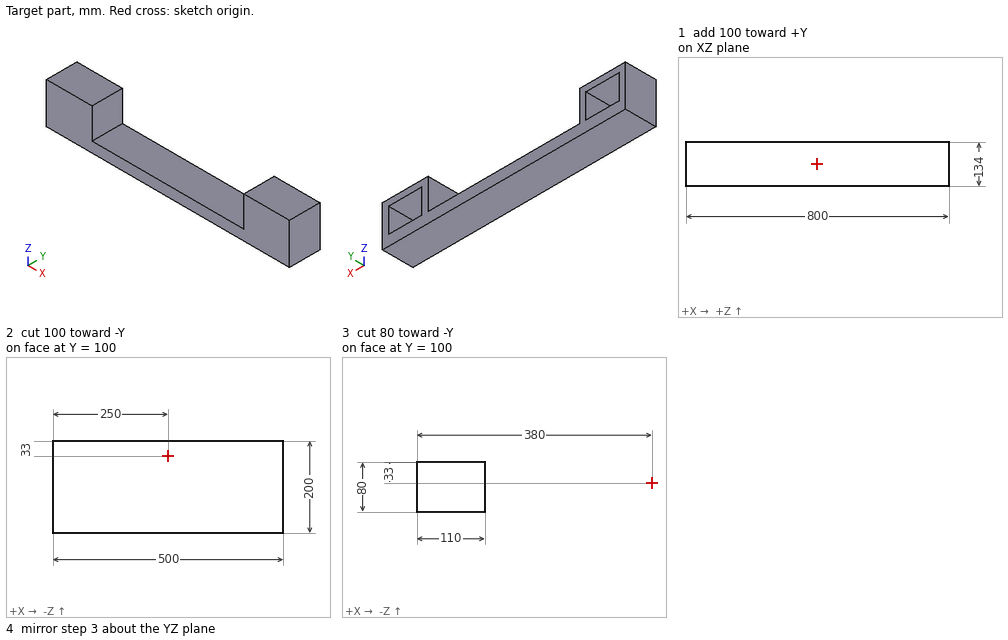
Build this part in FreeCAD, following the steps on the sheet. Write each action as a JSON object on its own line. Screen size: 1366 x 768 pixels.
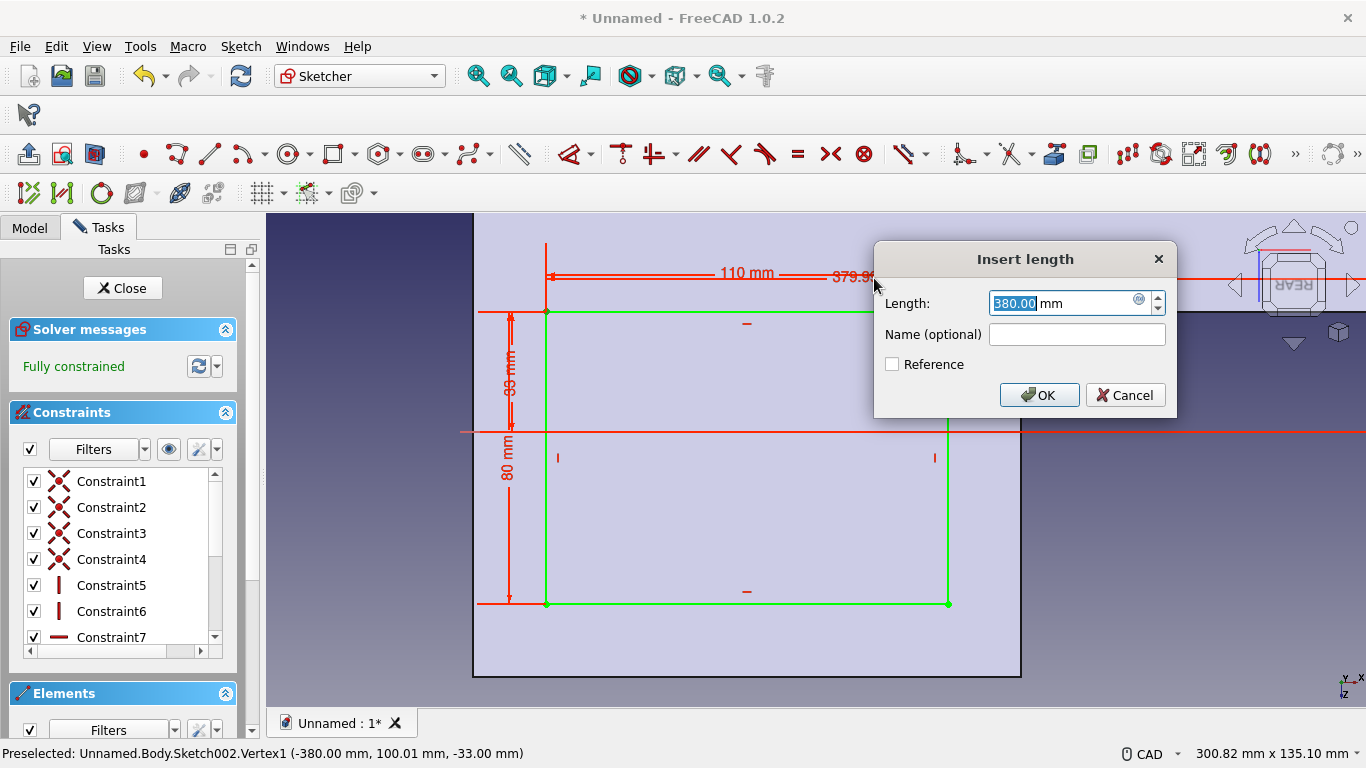
{"action": "type", "text": "380"}
{"action": "key", "text": "Return"}
{"action": "key", "text": "Escape"}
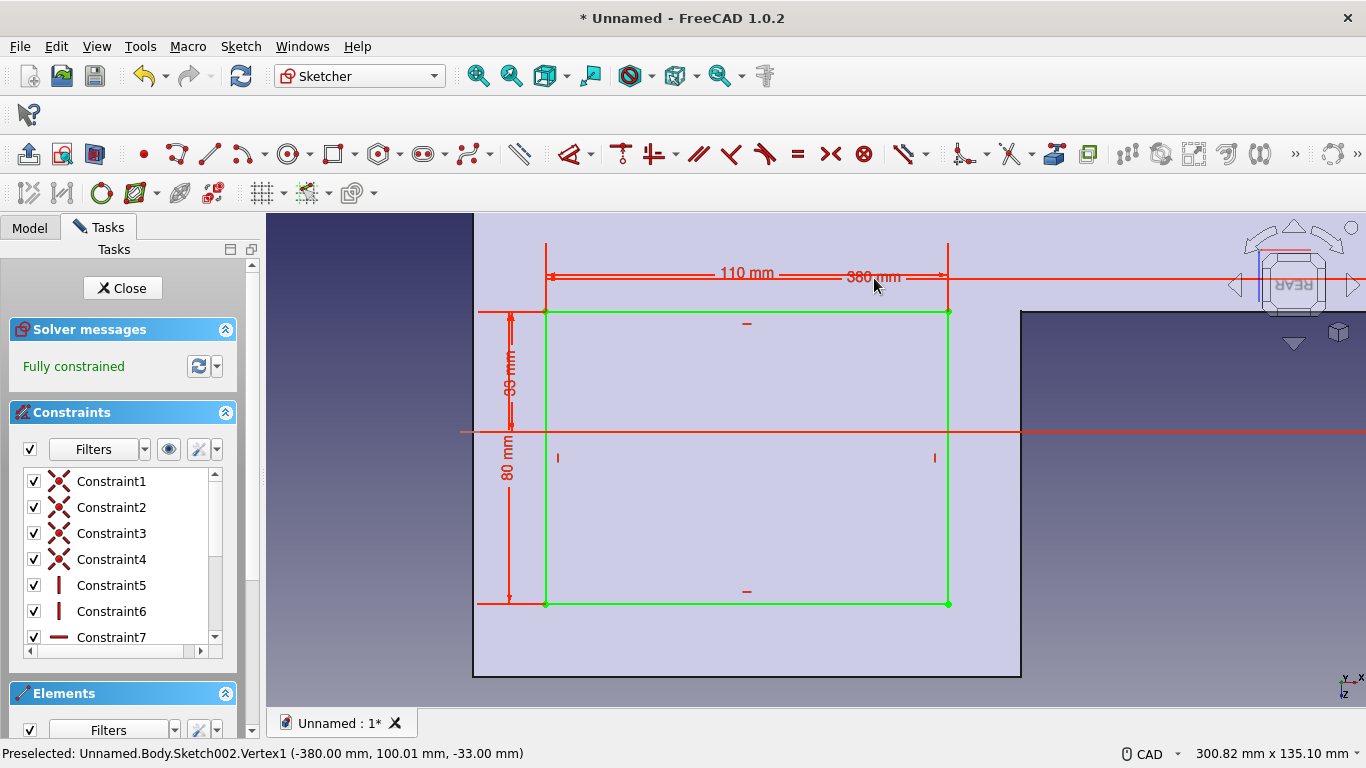
{"action": "left_click", "coordinate": [123, 288]}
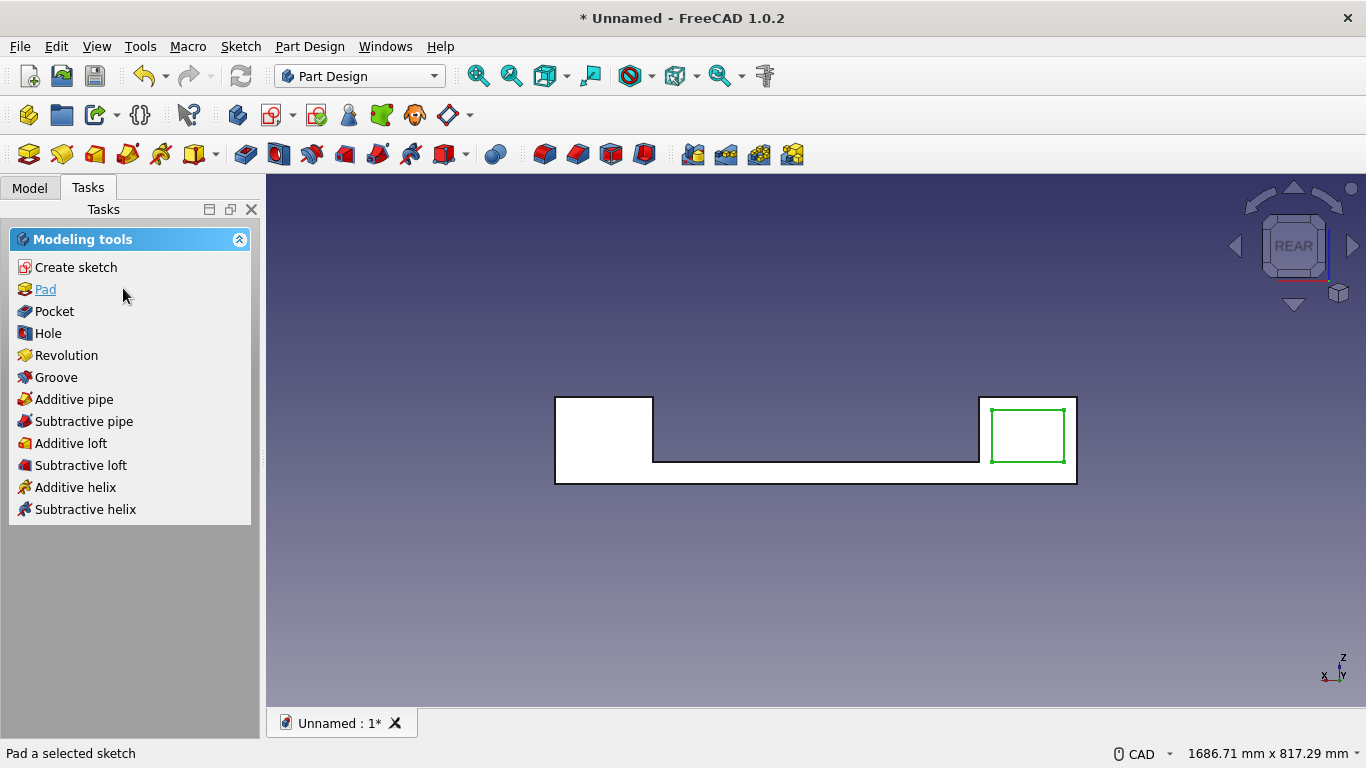
{"action": "left_click", "coordinate": [246, 154]}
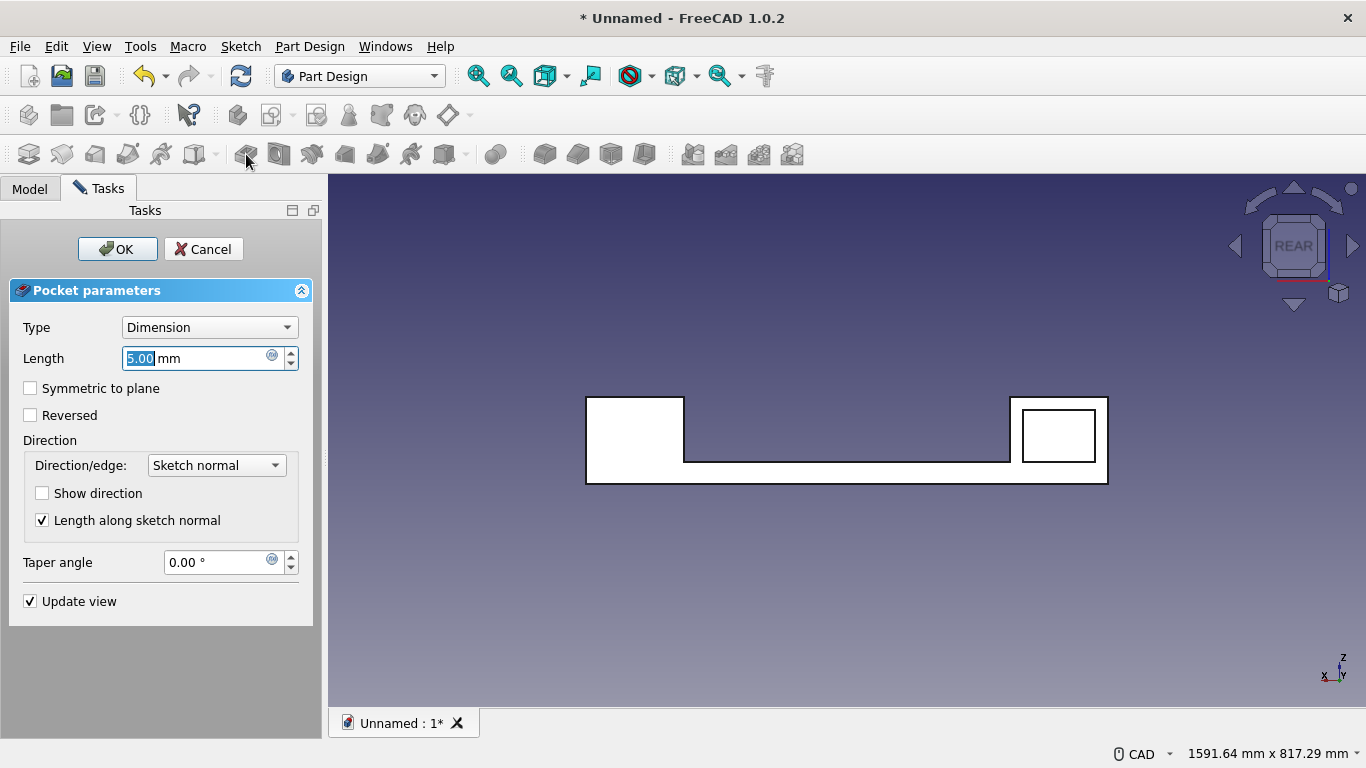
{"action": "type", "text": "80"}
{"action": "key", "text": "Tab"}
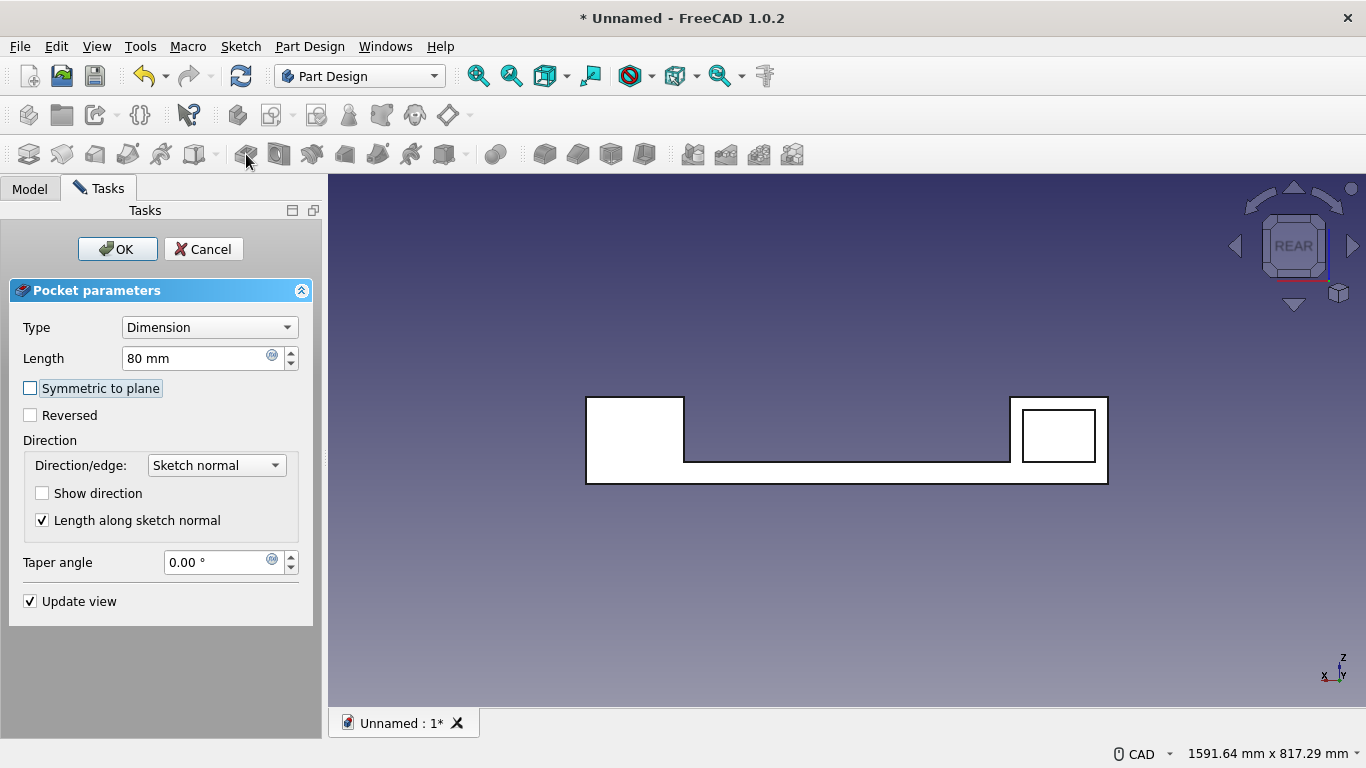
{"action": "left_click", "coordinate": [118, 249]}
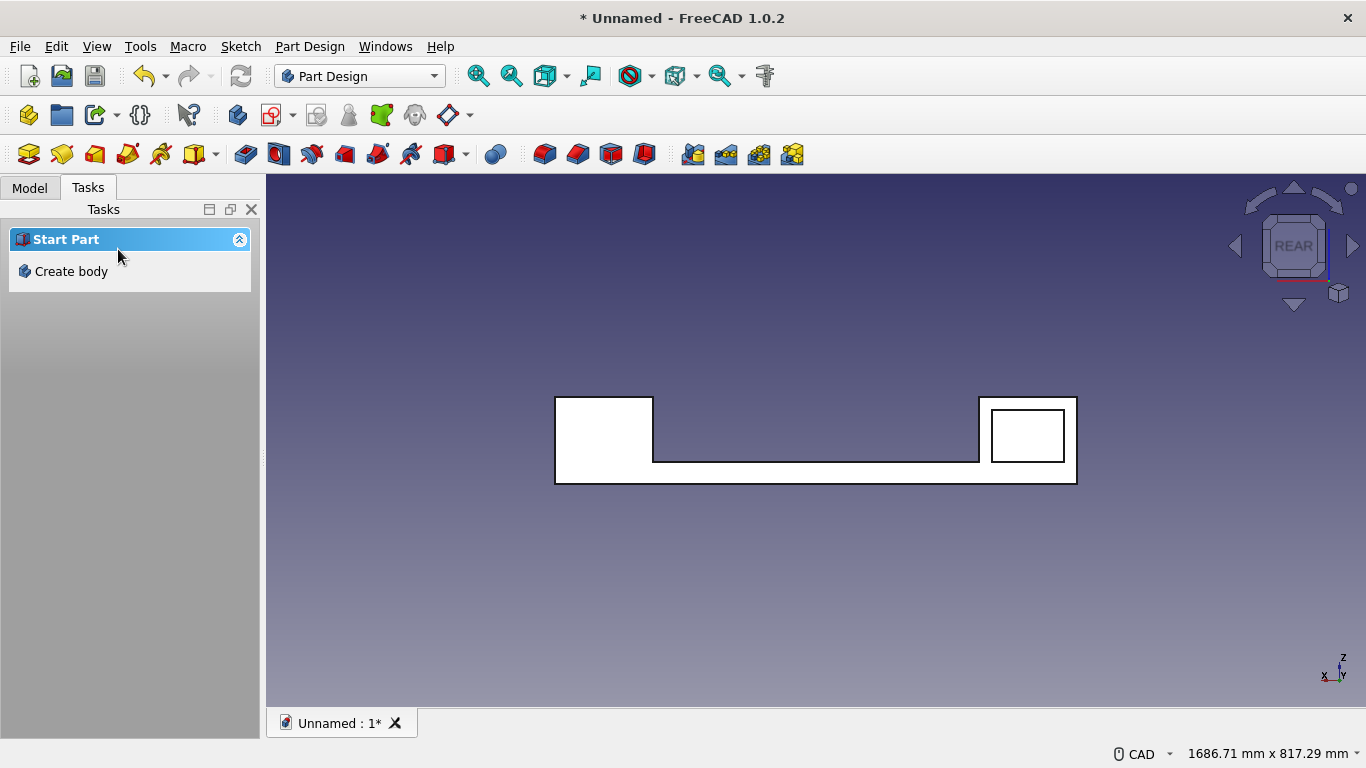
{"action": "left_click", "coordinate": [30, 188]}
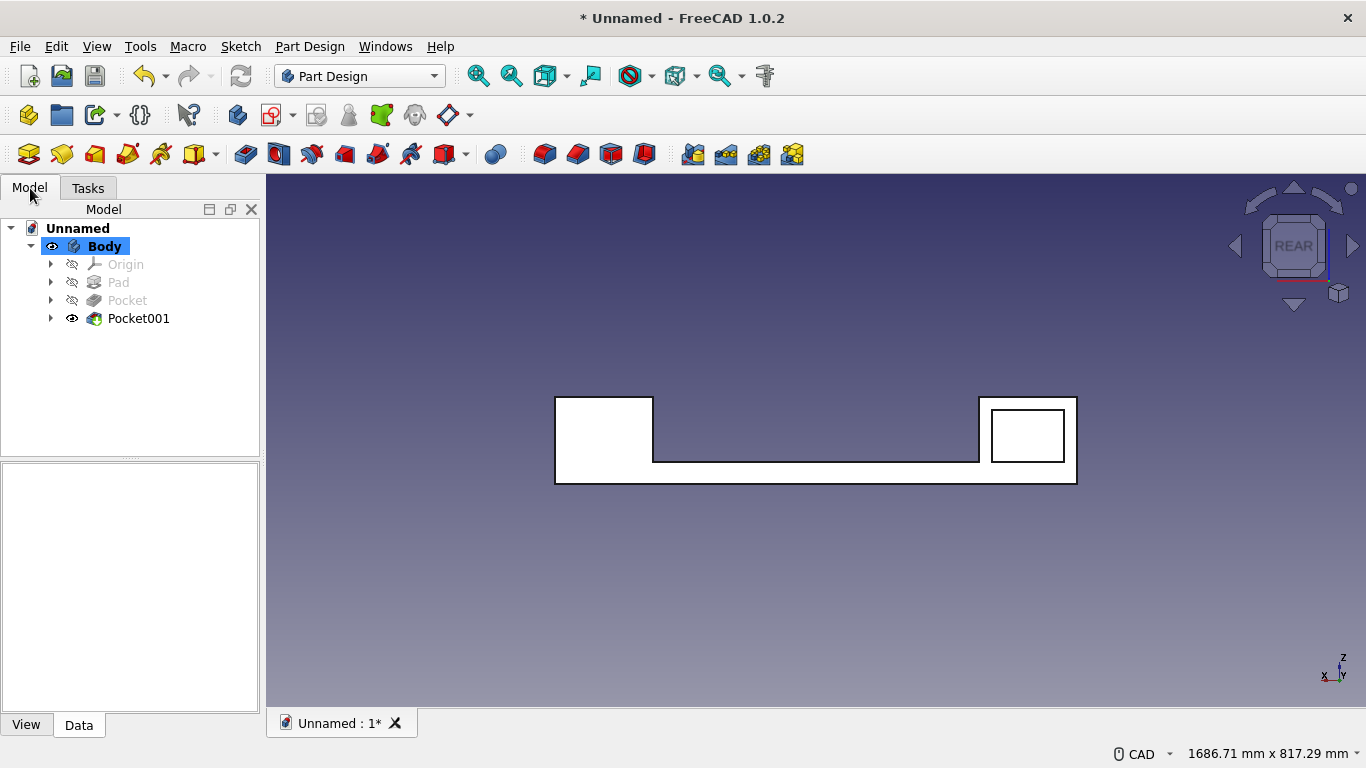
{"action": "left_click", "coordinate": [117, 318]}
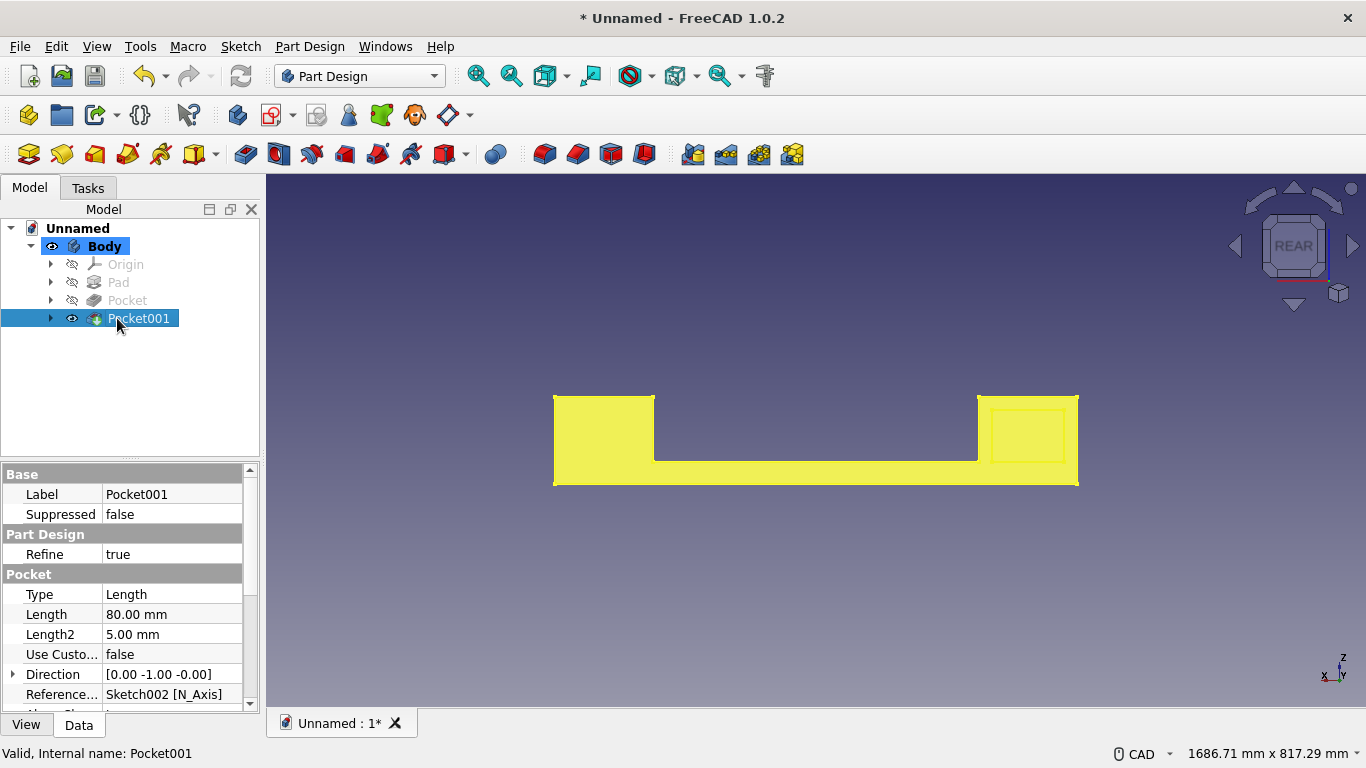
{"action": "left_click", "coordinate": [693, 154]}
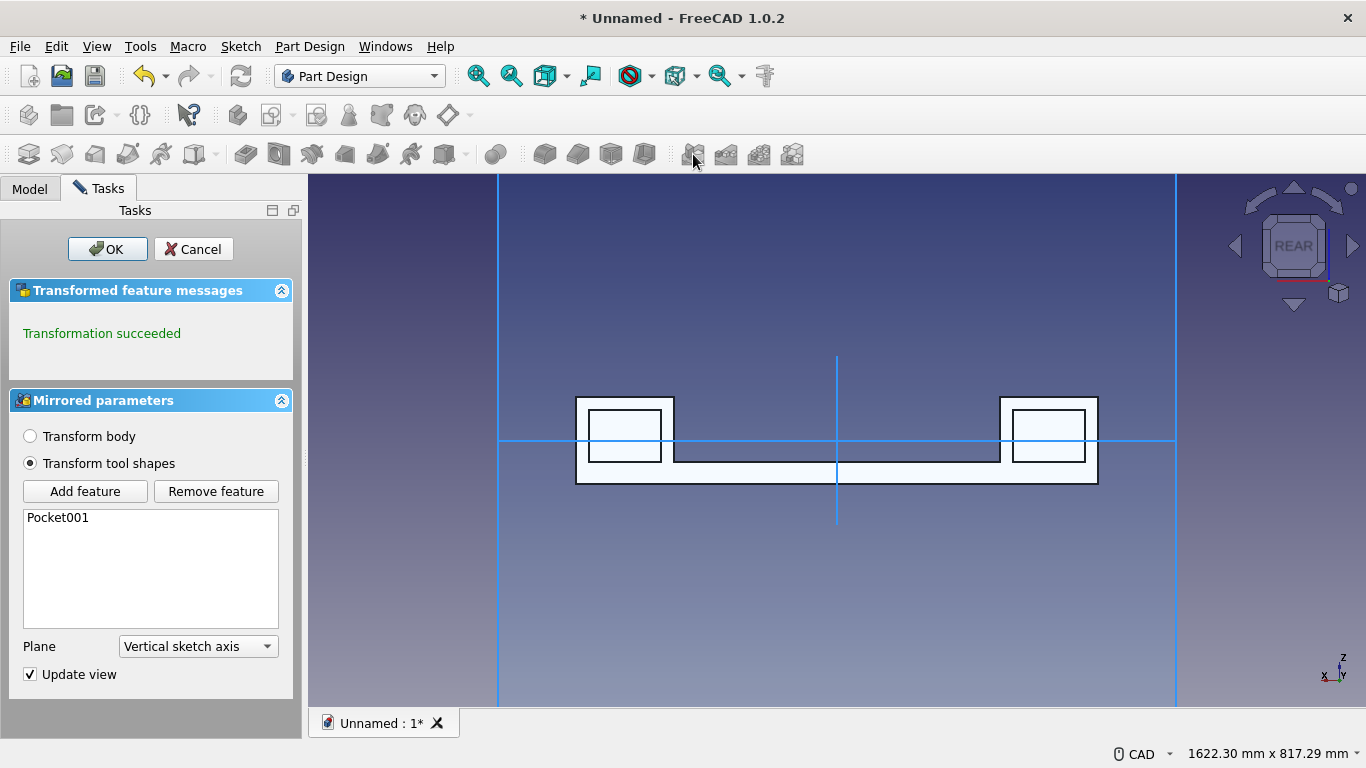
{"action": "left_click", "coordinate": [199, 646]}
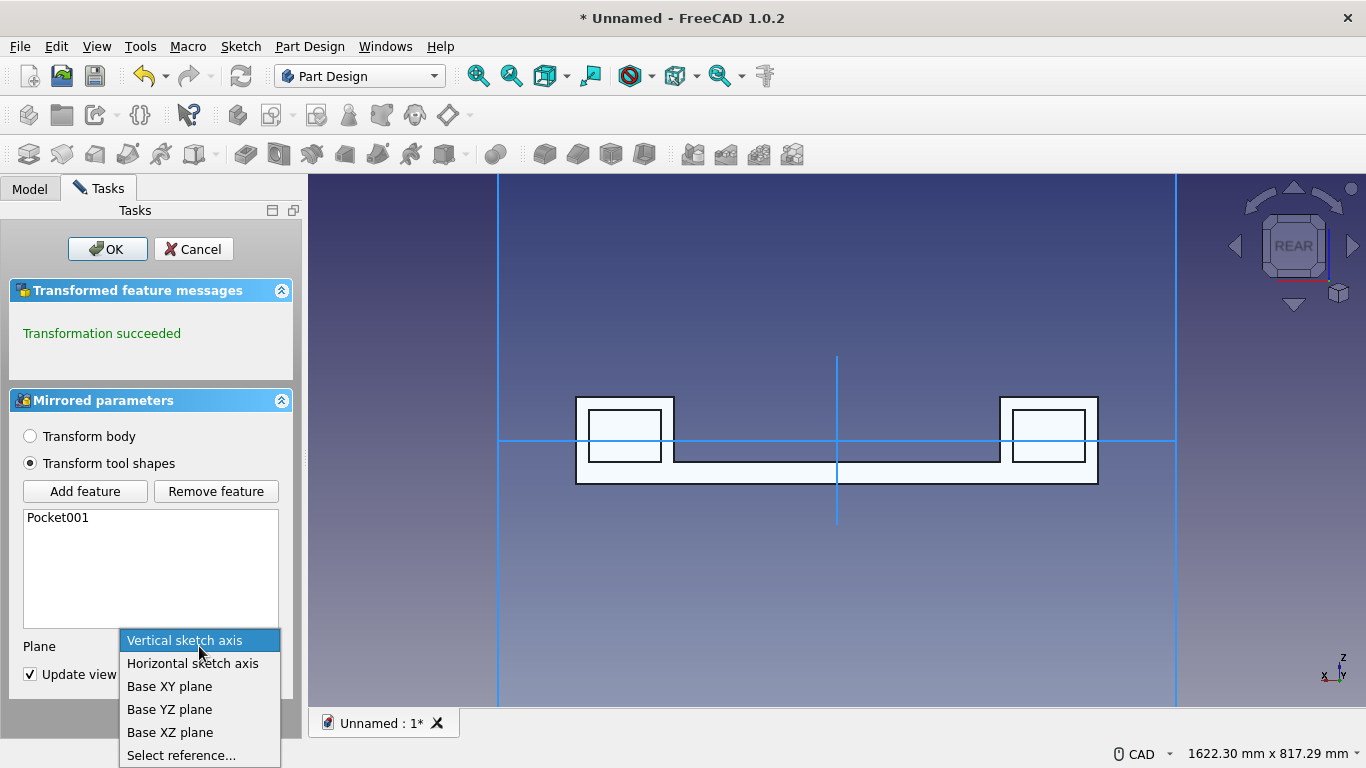
{"action": "left_click", "coordinate": [198, 710]}